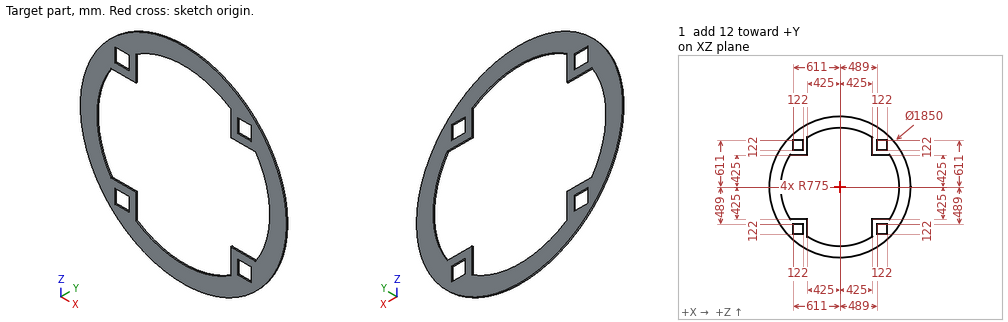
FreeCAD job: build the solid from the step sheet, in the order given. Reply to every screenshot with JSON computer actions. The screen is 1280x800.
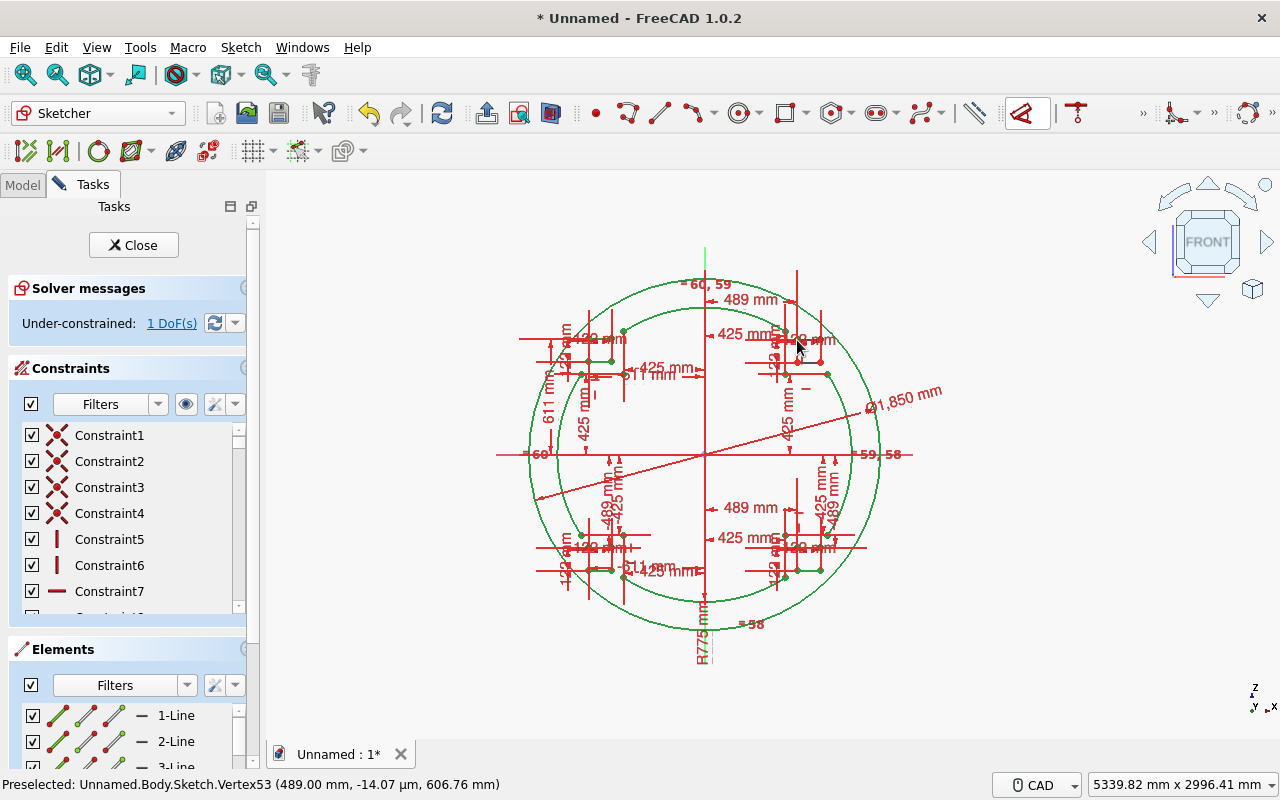
{"action": "left_click", "coordinate": [1044, 114]}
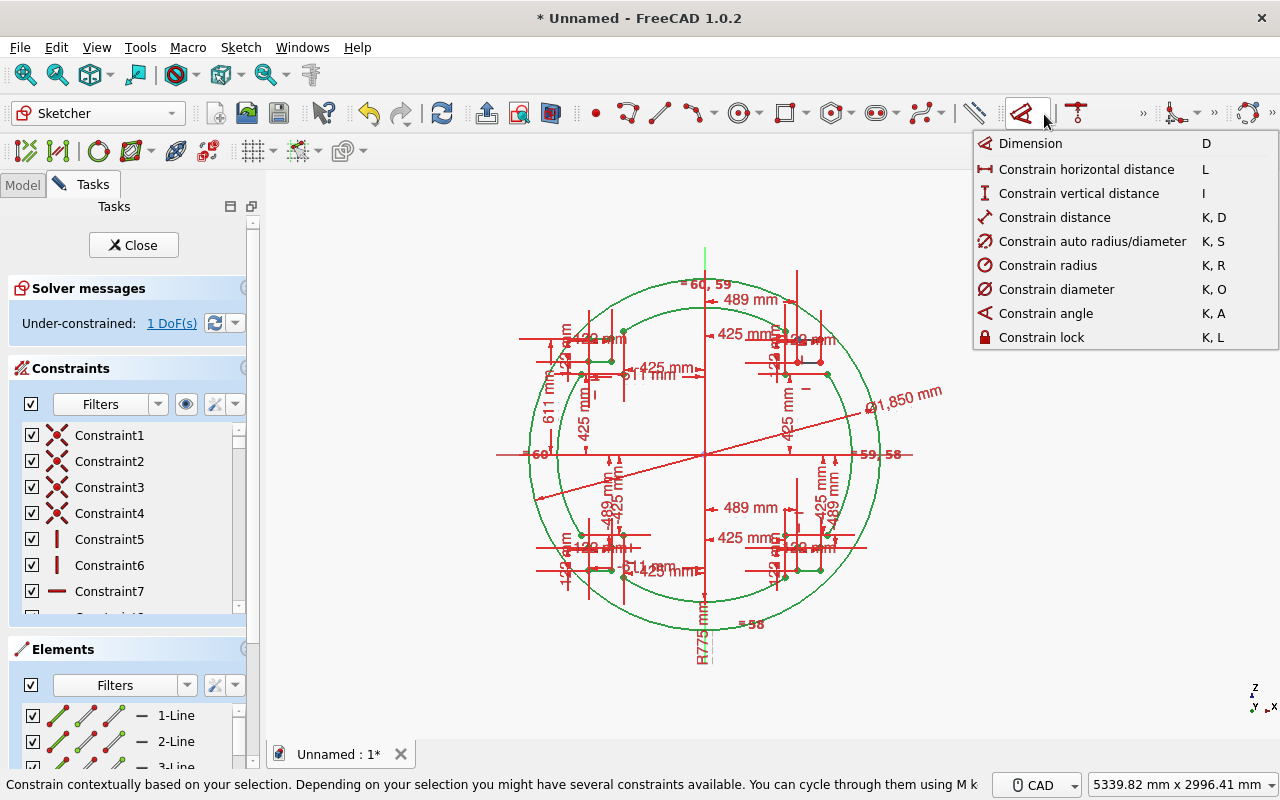
{"action": "left_click", "coordinate": [1126, 193]}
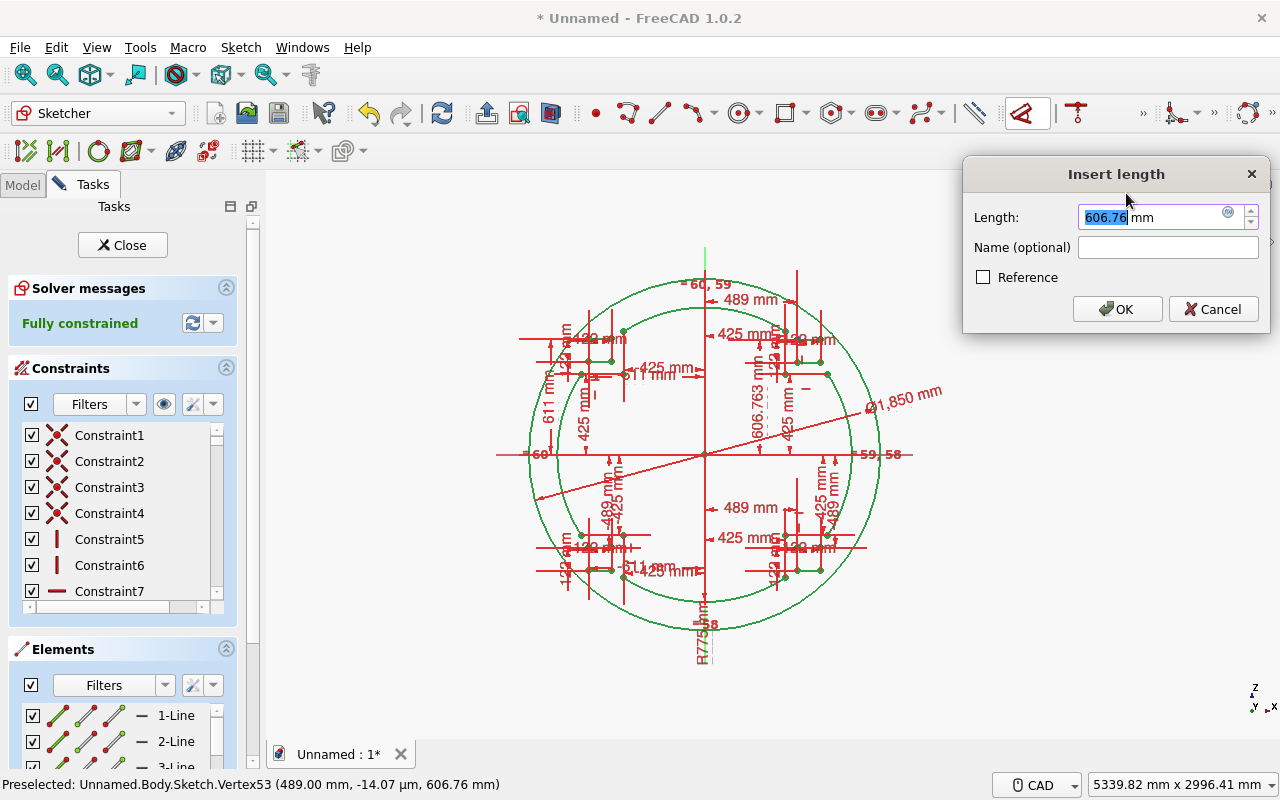
{"action": "type", "text": "611"}
{"action": "key", "text": "Return"}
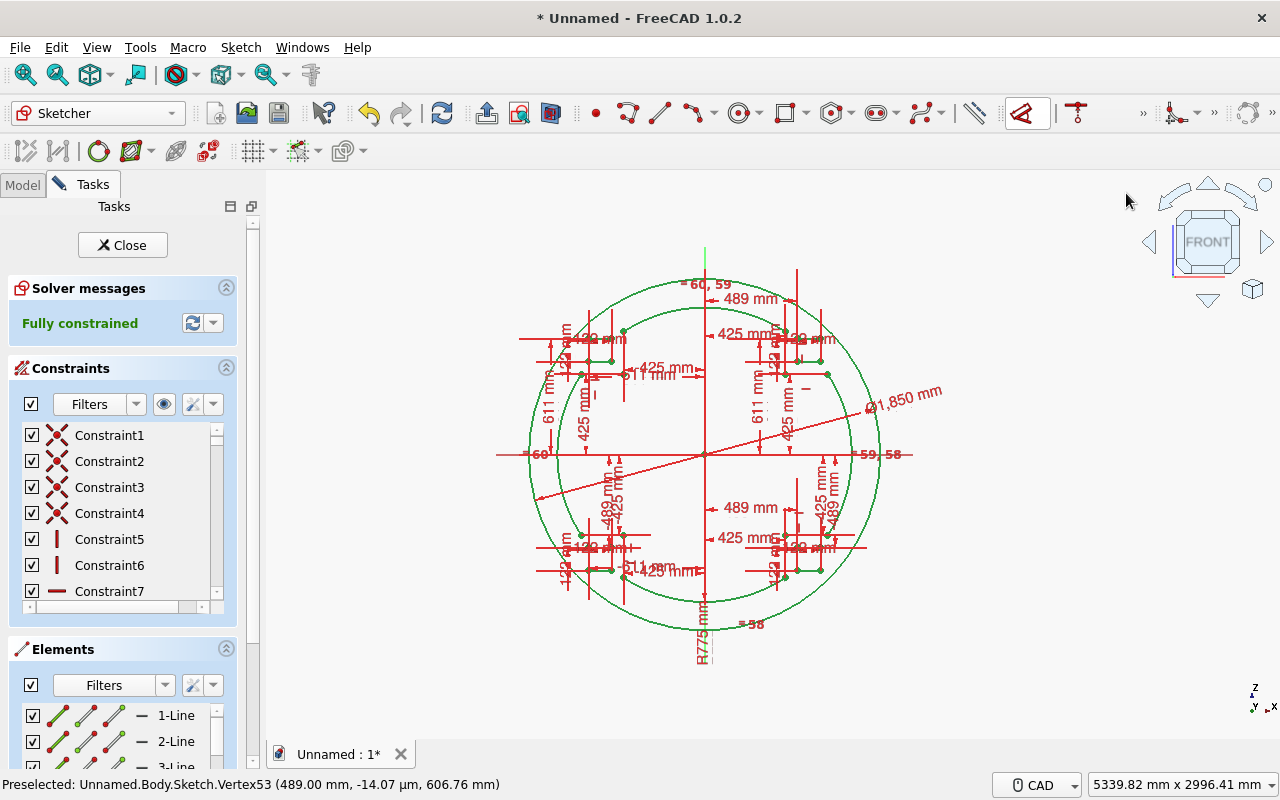
{"action": "left_click", "coordinate": [123, 245]}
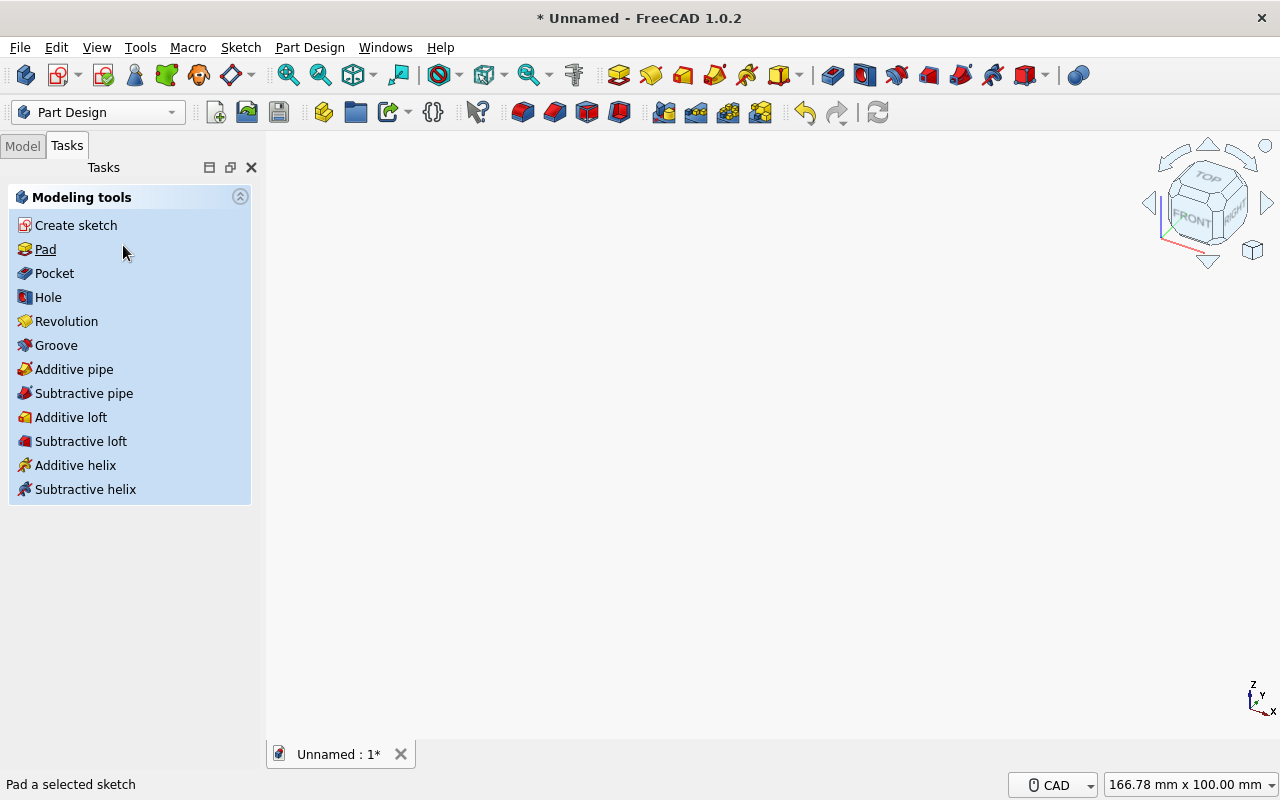
{"action": "left_click", "coordinate": [620, 76]}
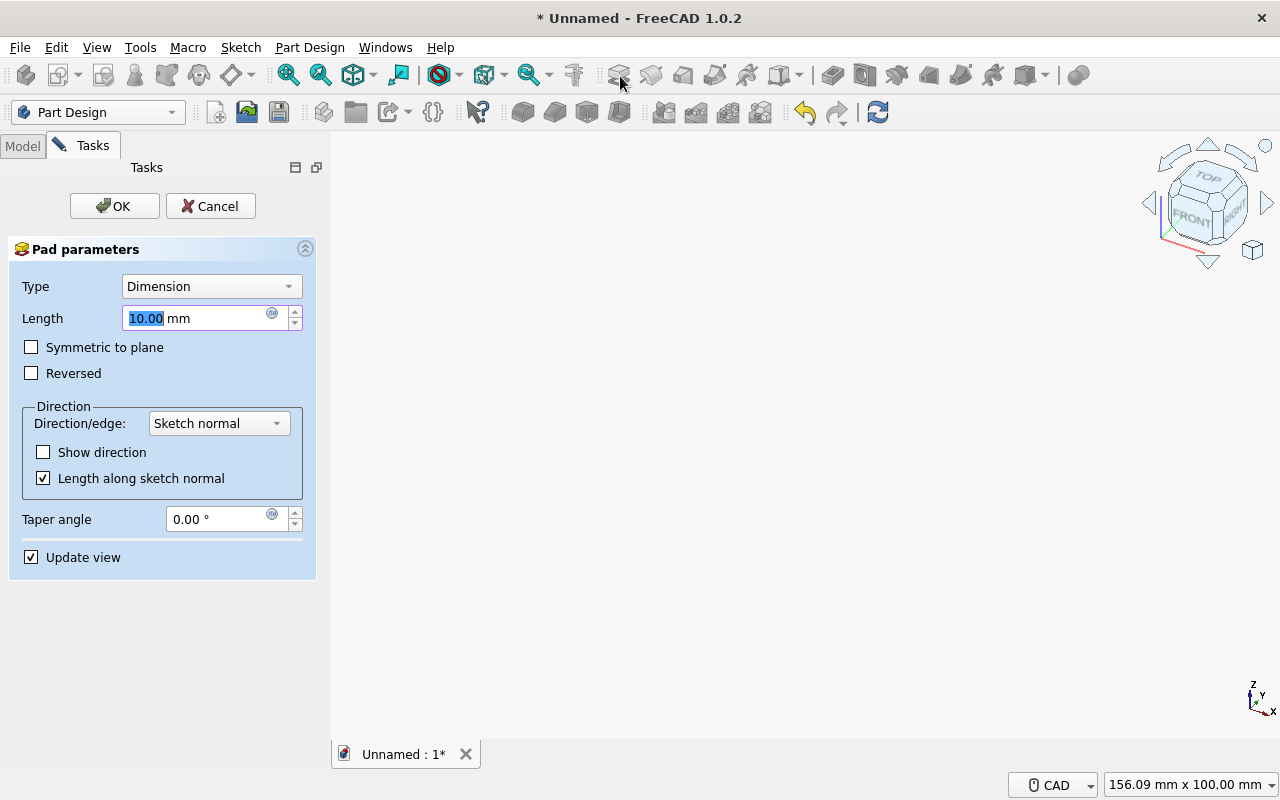
{"action": "type", "text": "12"}
{"action": "key", "text": "Tab"}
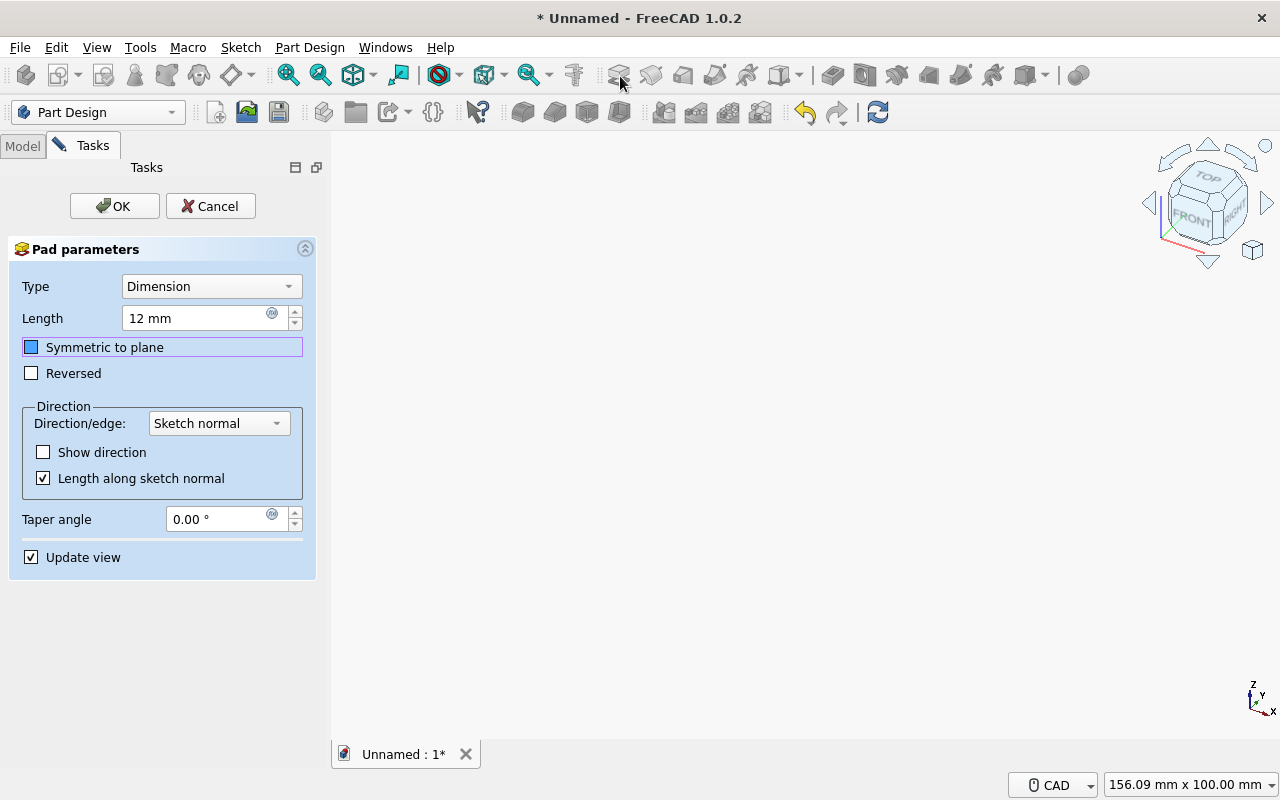
{"action": "left_click", "coordinate": [30, 373]}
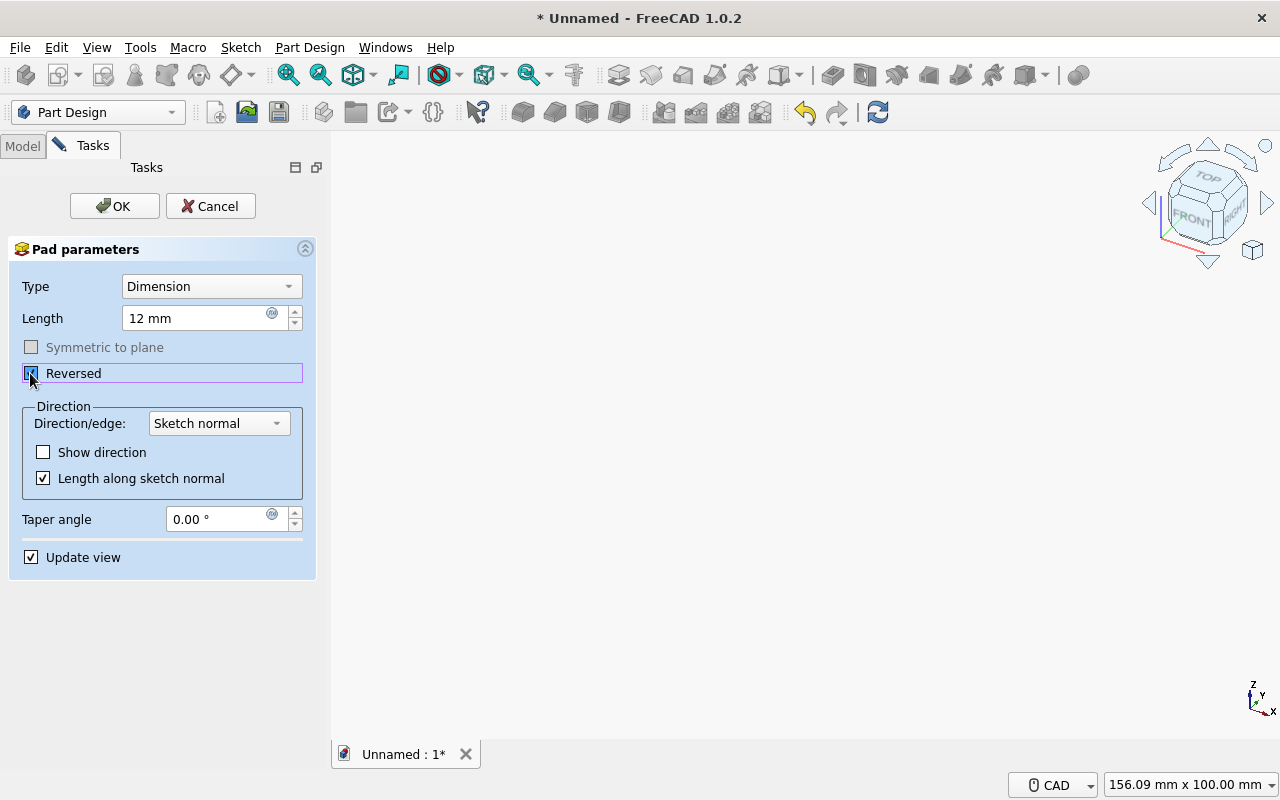
{"action": "left_click", "coordinate": [115, 206]}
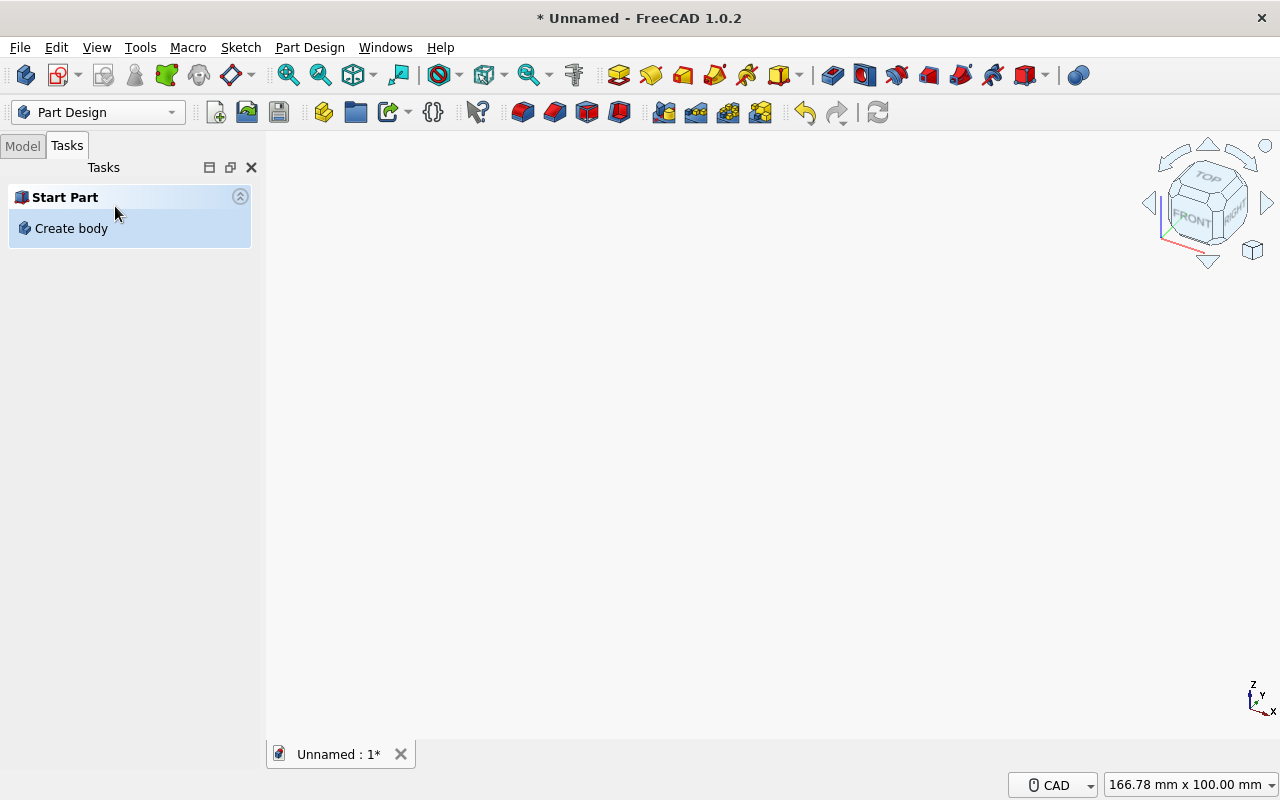
{"action": "key", "text": "0"}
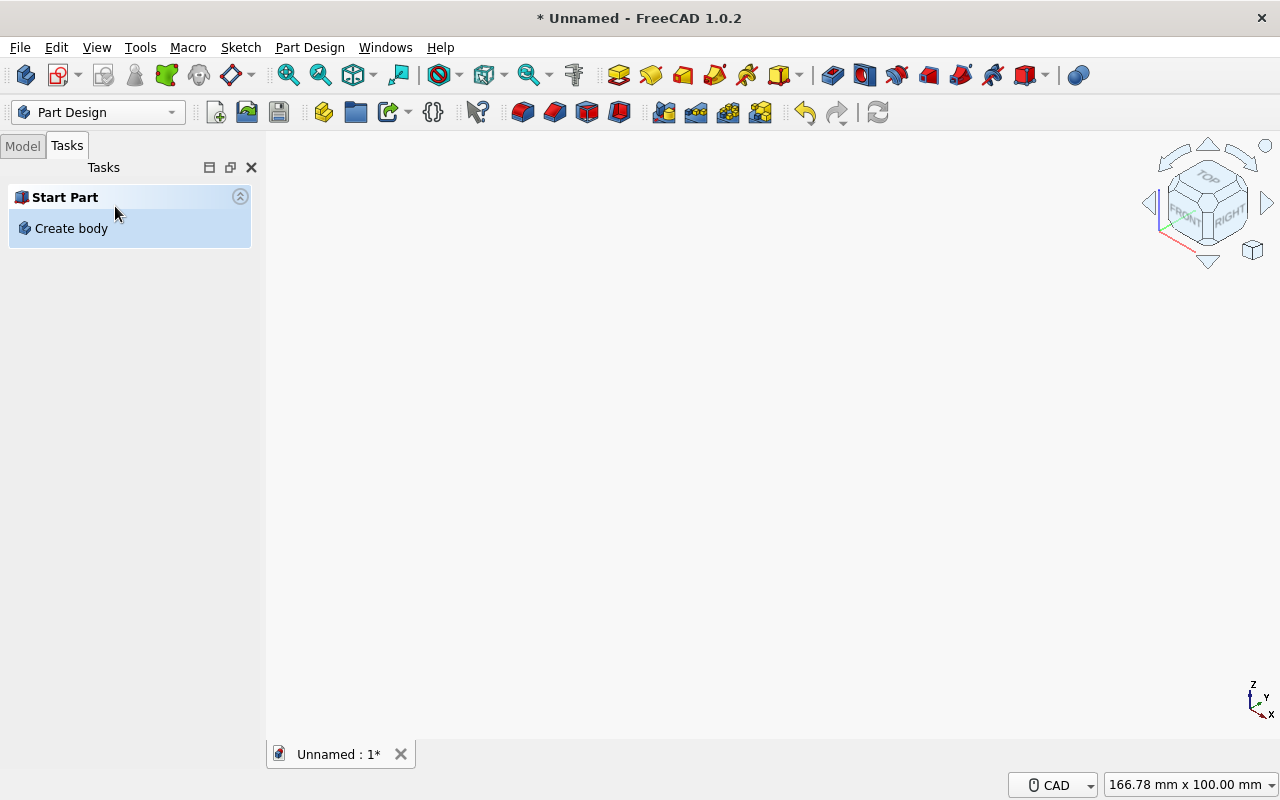
{"action": "key", "text": "v f"}